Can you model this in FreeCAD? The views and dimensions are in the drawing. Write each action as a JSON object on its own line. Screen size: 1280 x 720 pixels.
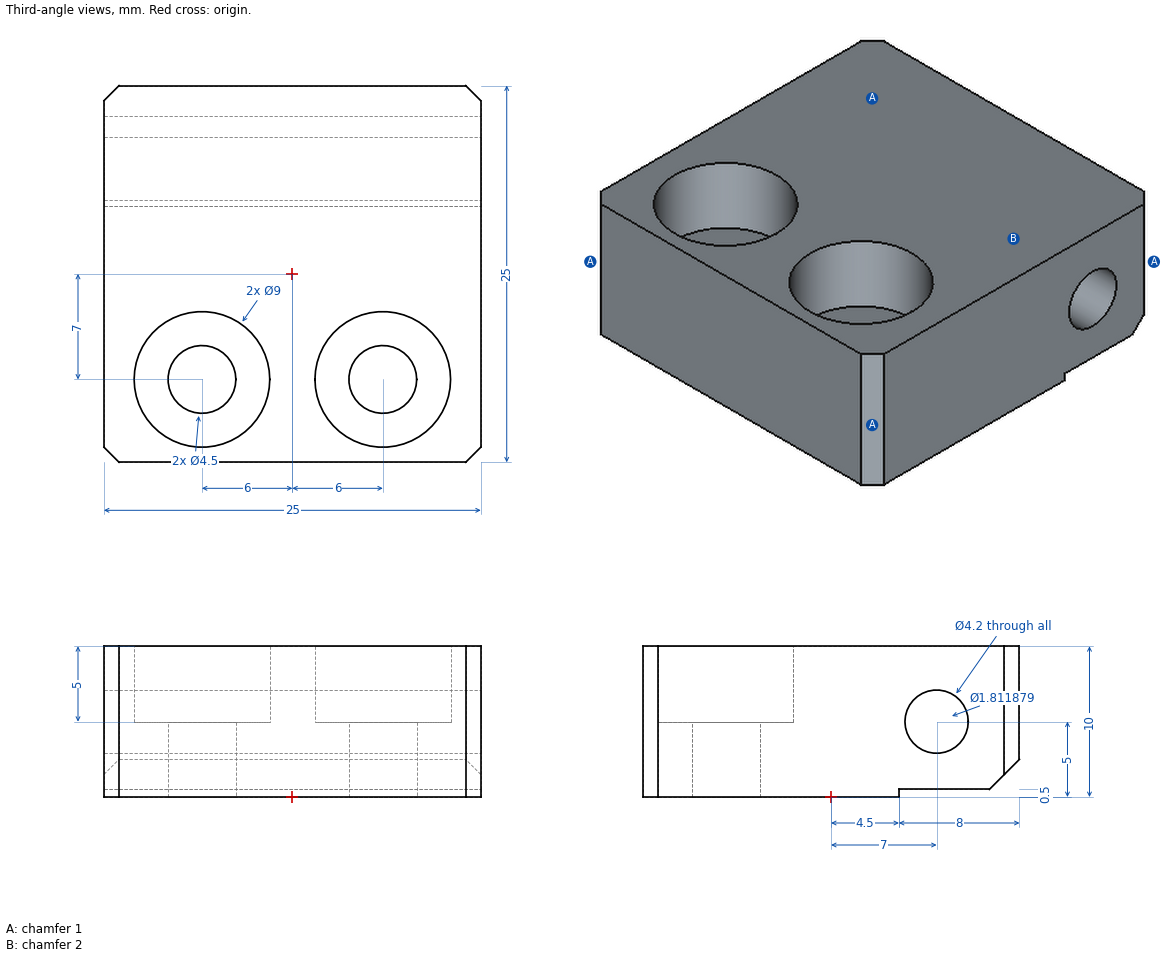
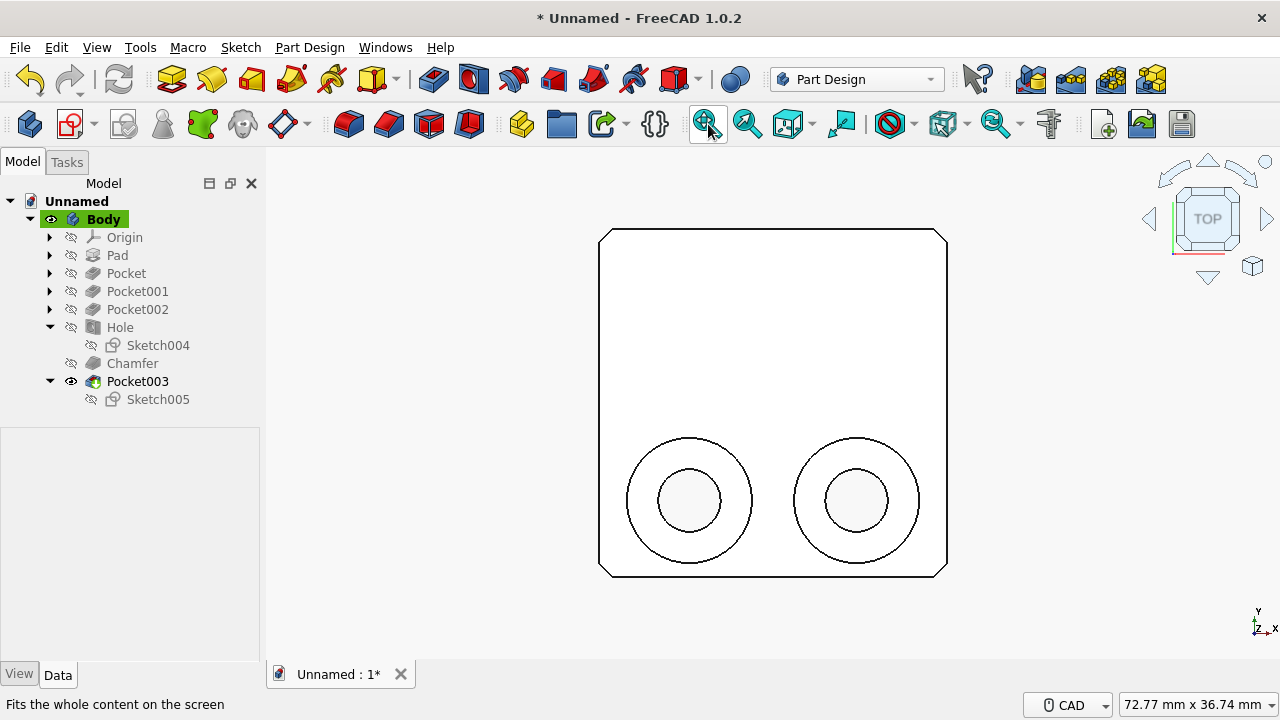
{"action": "key", "text": "1"}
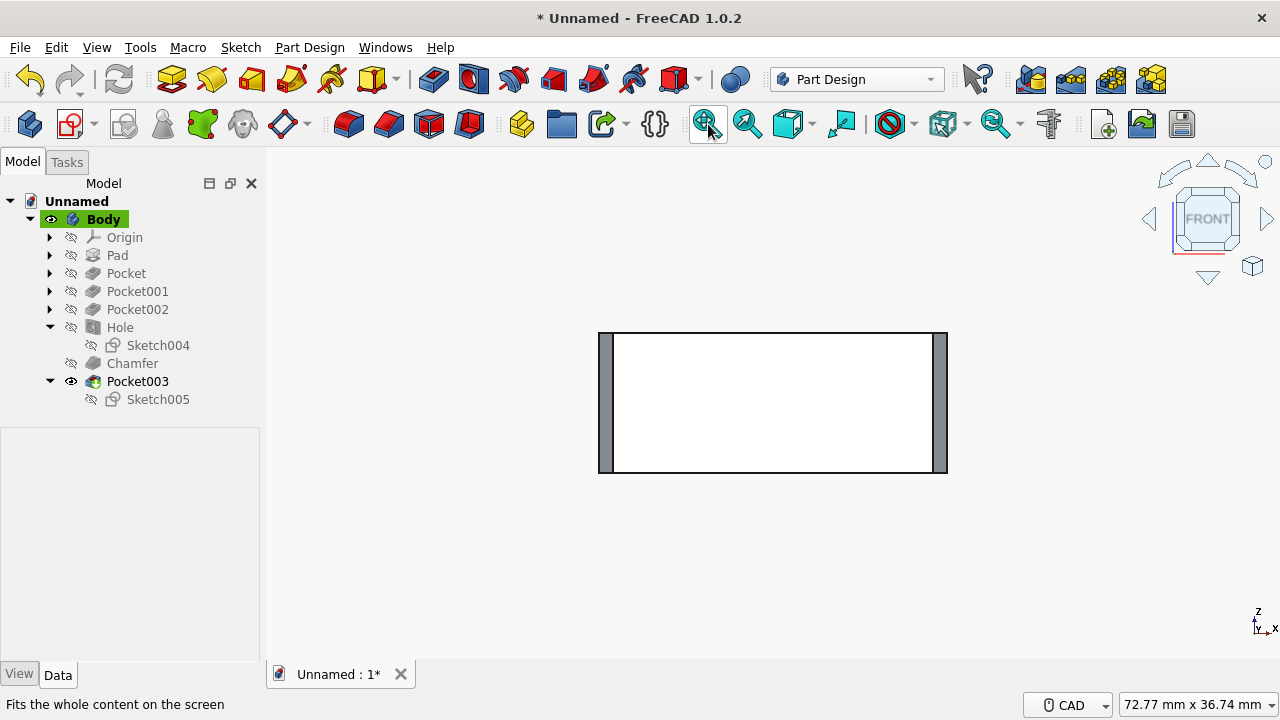
{"action": "key", "text": "v f"}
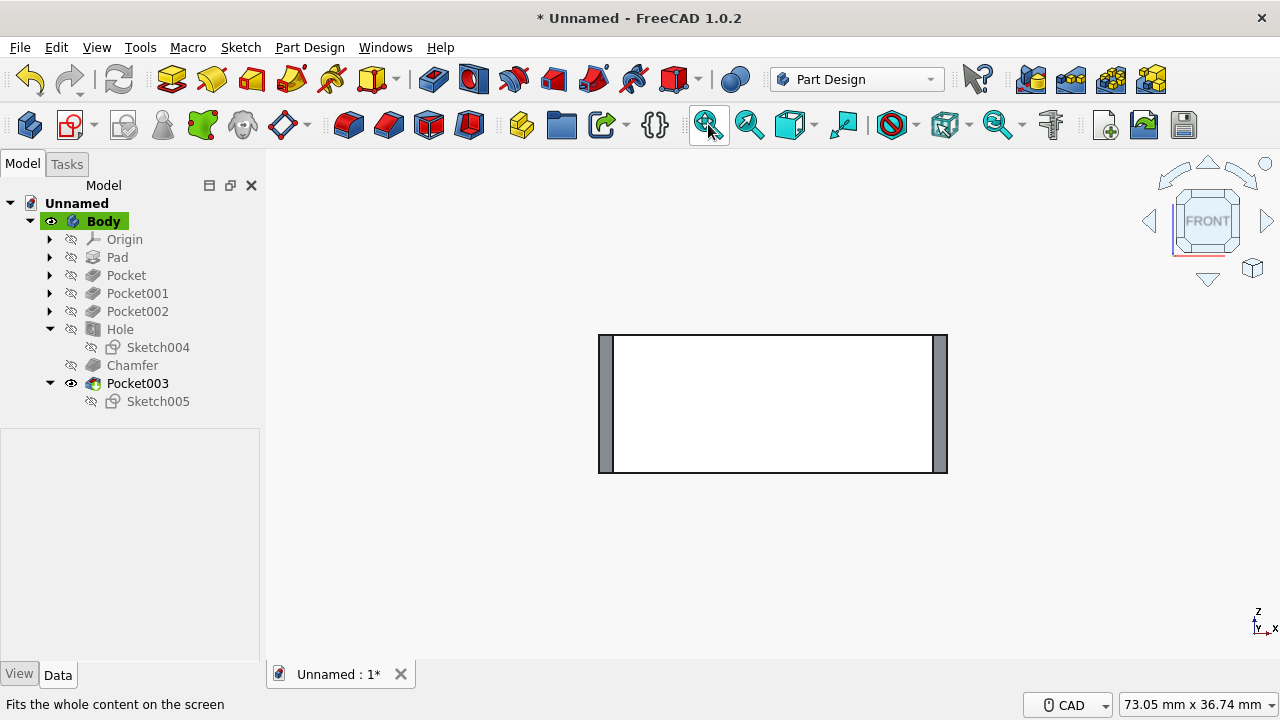
{"action": "key", "text": "3"}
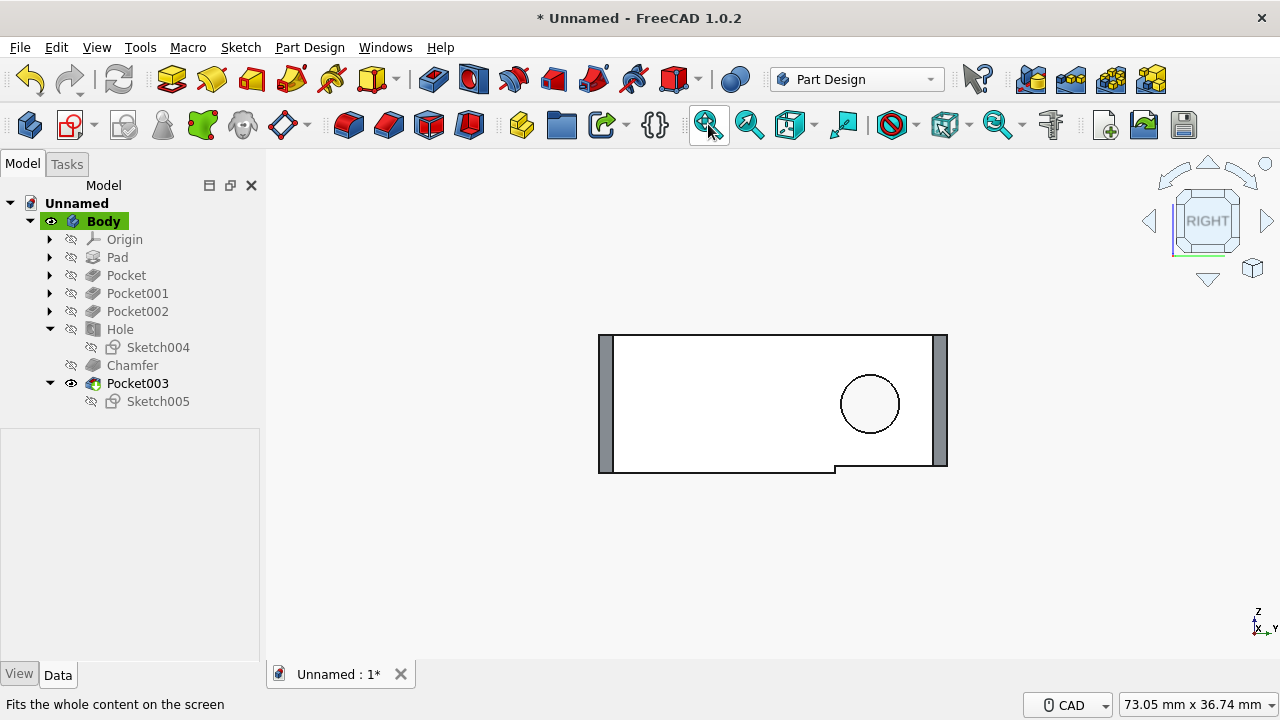
{"action": "left_click", "coordinate": [710, 126]}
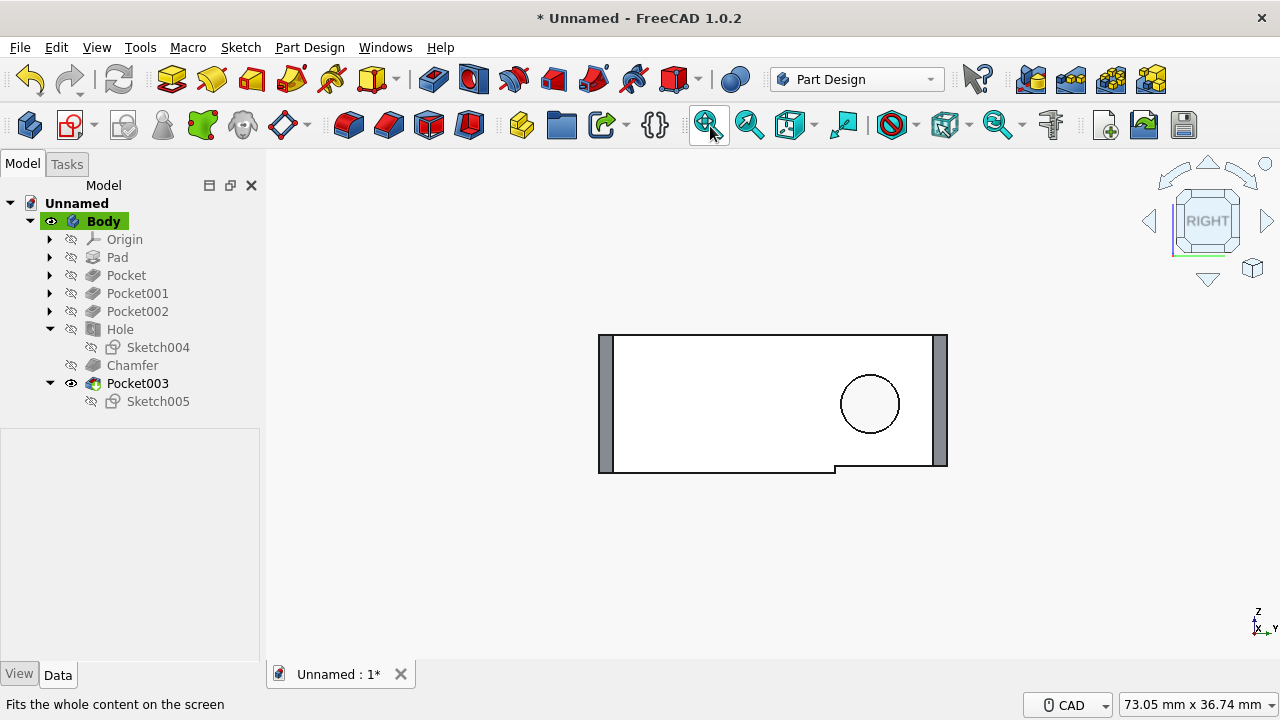
{"action": "key", "text": "5"}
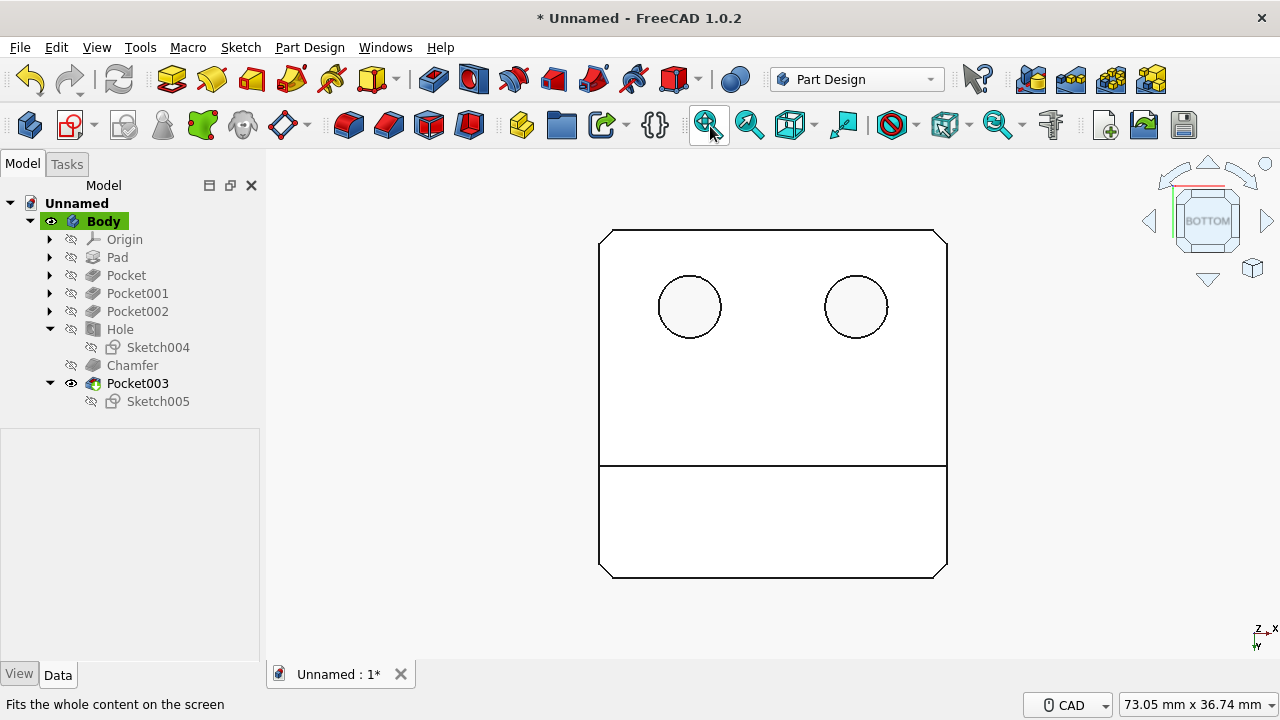
{"action": "left_click", "coordinate": [773, 577]}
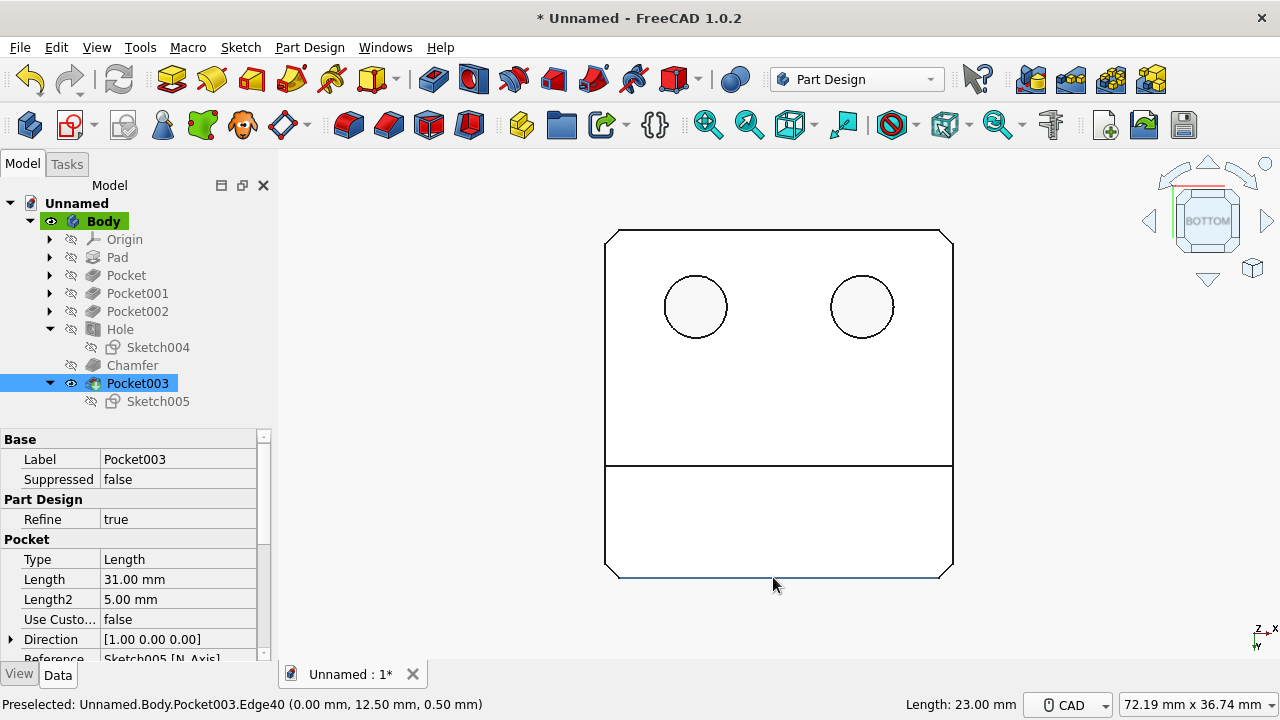
{"action": "left_click", "coordinate": [390, 126]}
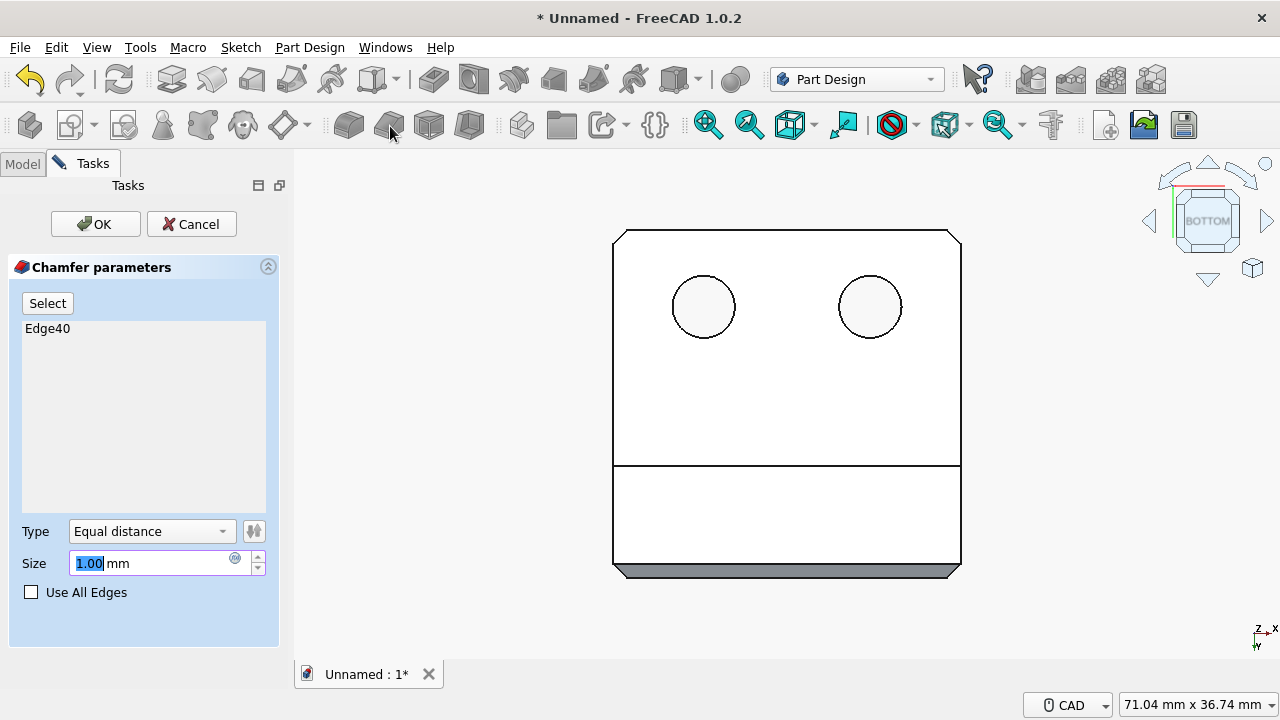
{"action": "type", "text": "2"}
{"action": "key", "text": "Tab"}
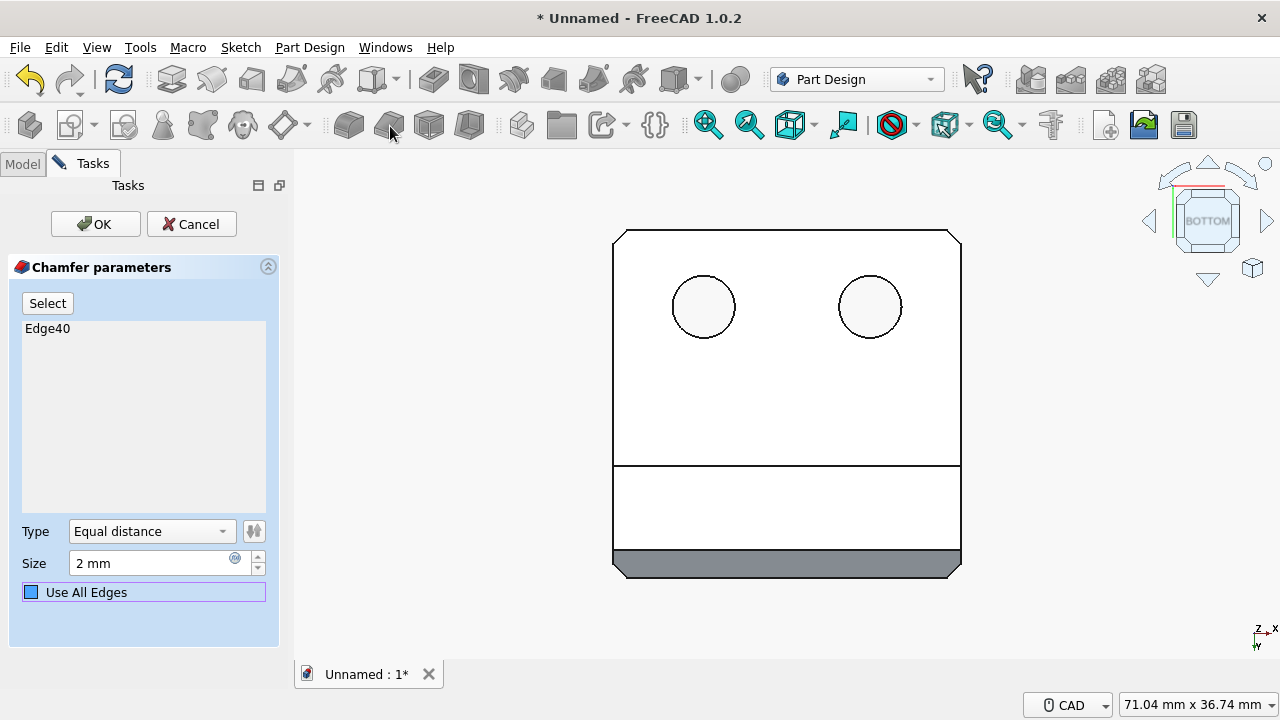
{"action": "left_click", "coordinate": [96, 224]}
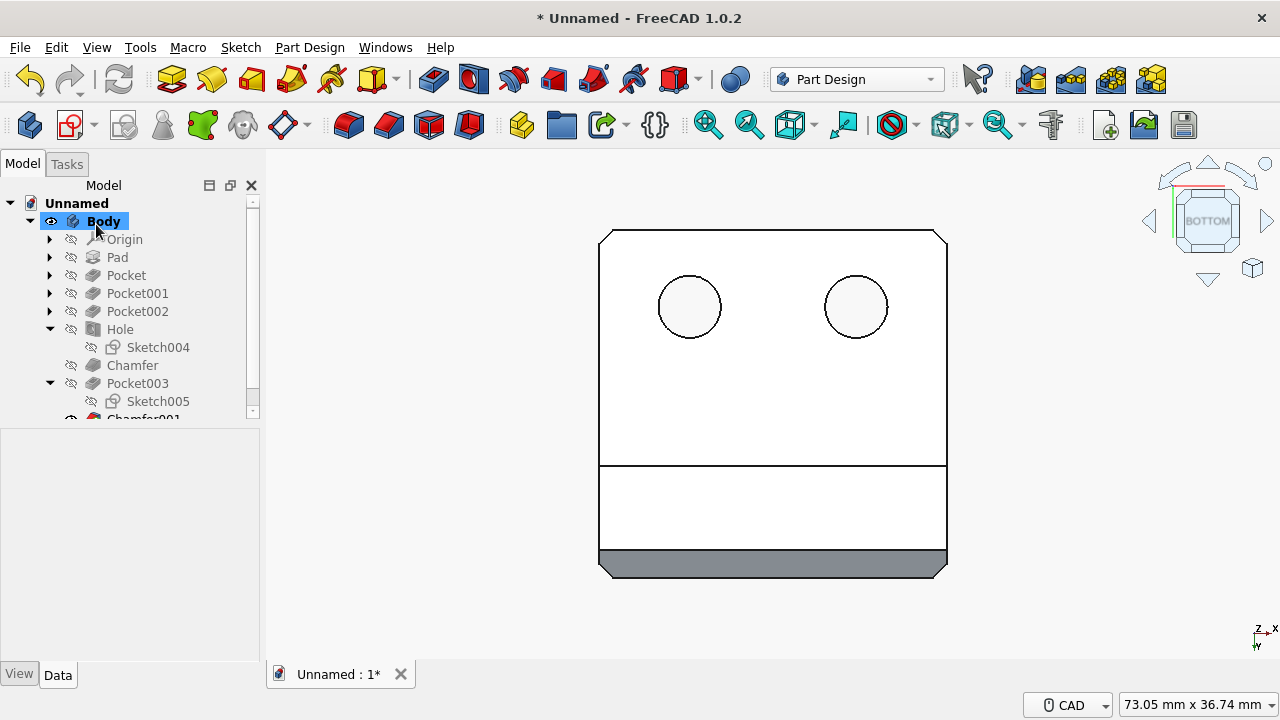
{"action": "key", "text": "0"}